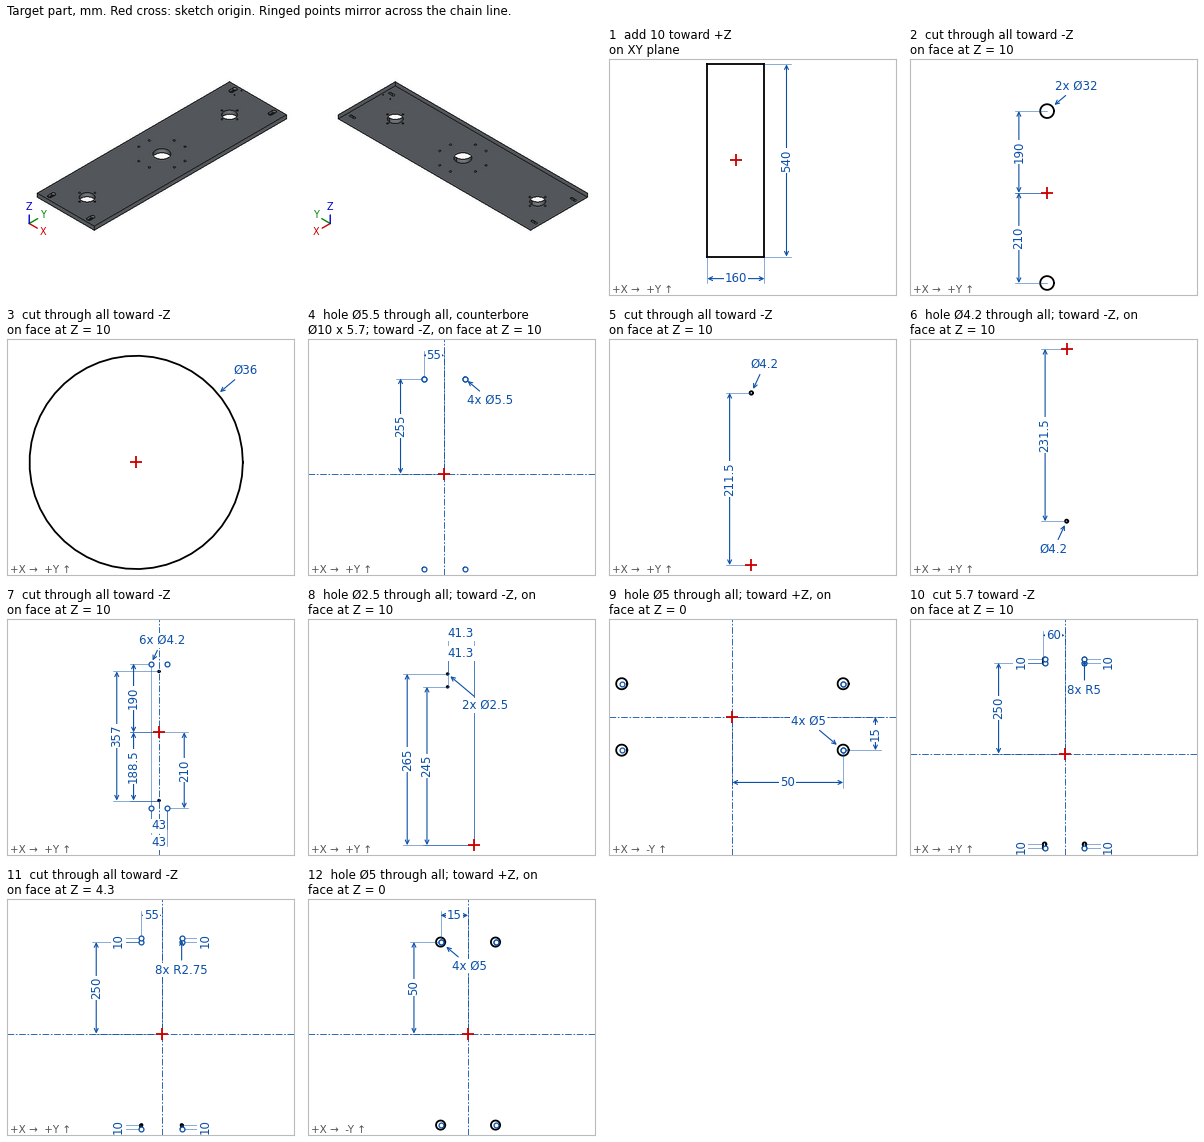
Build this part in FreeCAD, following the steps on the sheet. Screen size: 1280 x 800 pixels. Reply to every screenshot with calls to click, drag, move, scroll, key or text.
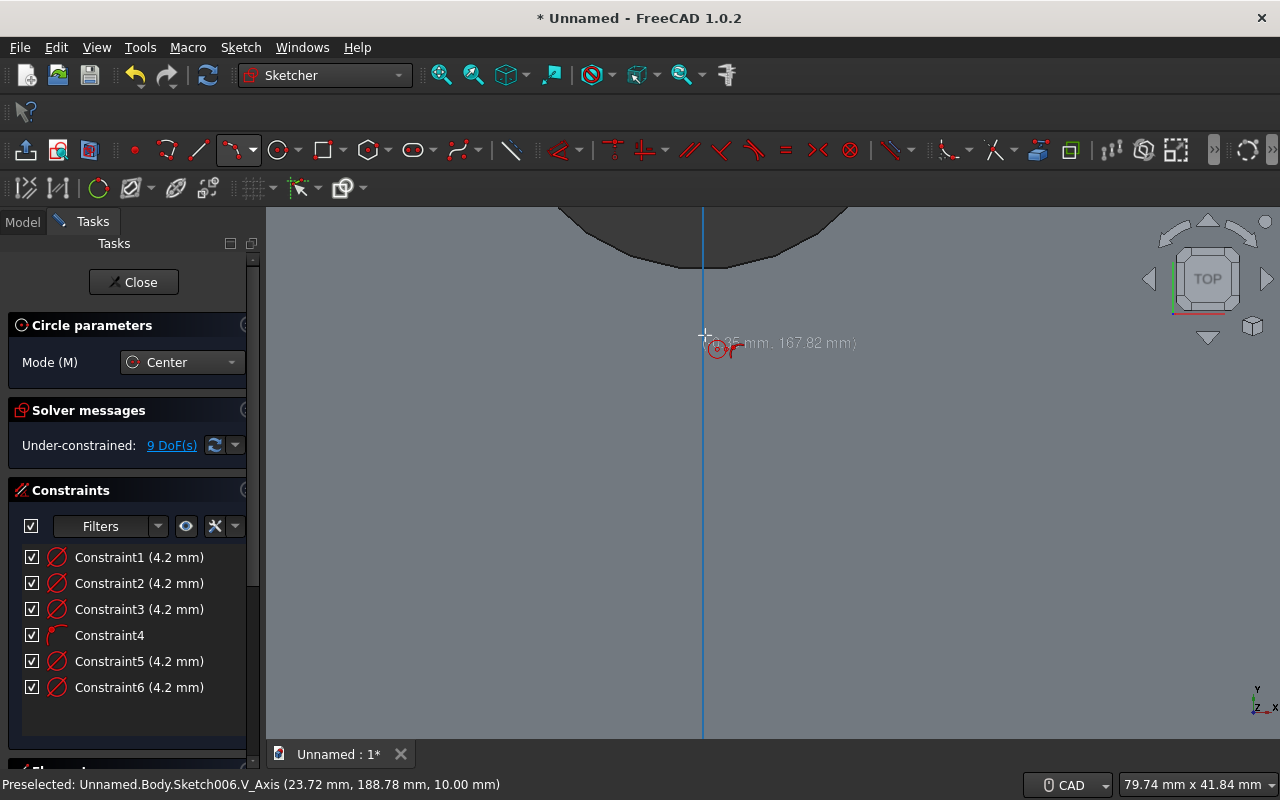
scroll(705, 335, down, 14)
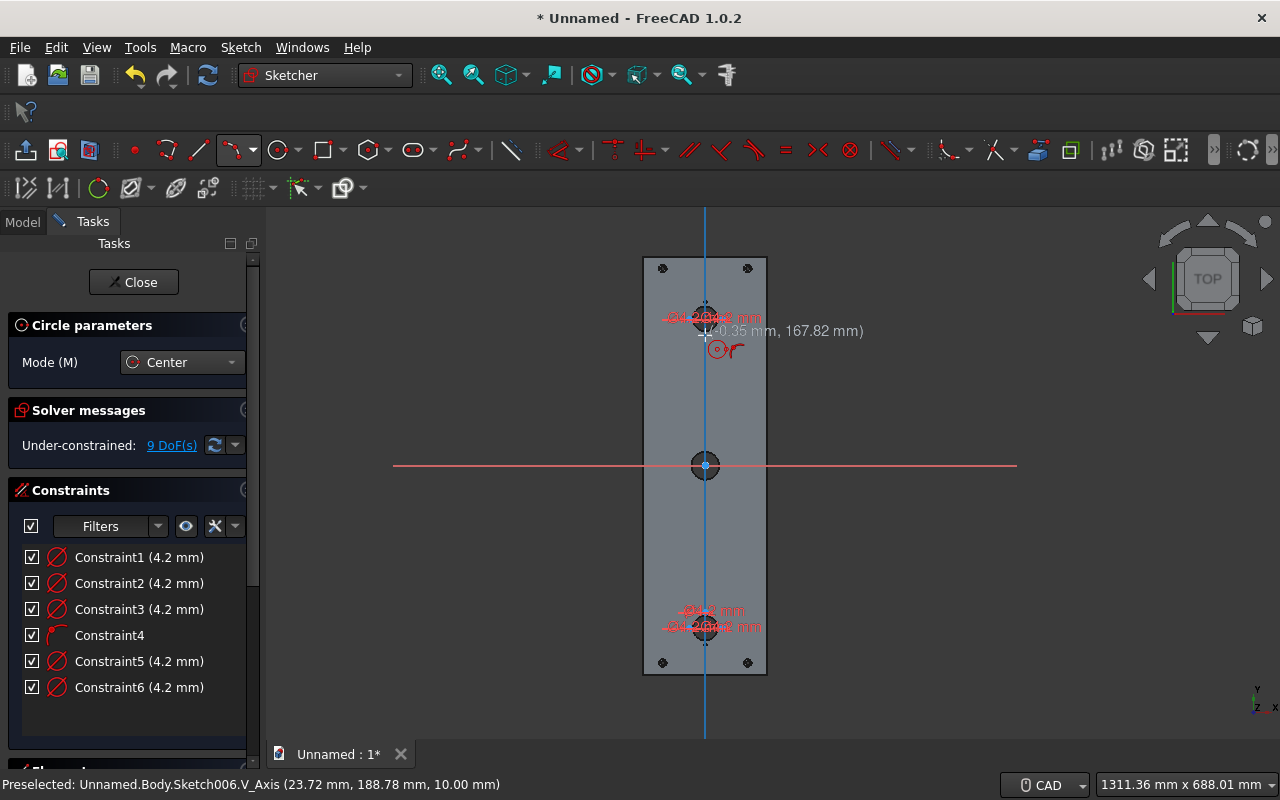
click(705, 335)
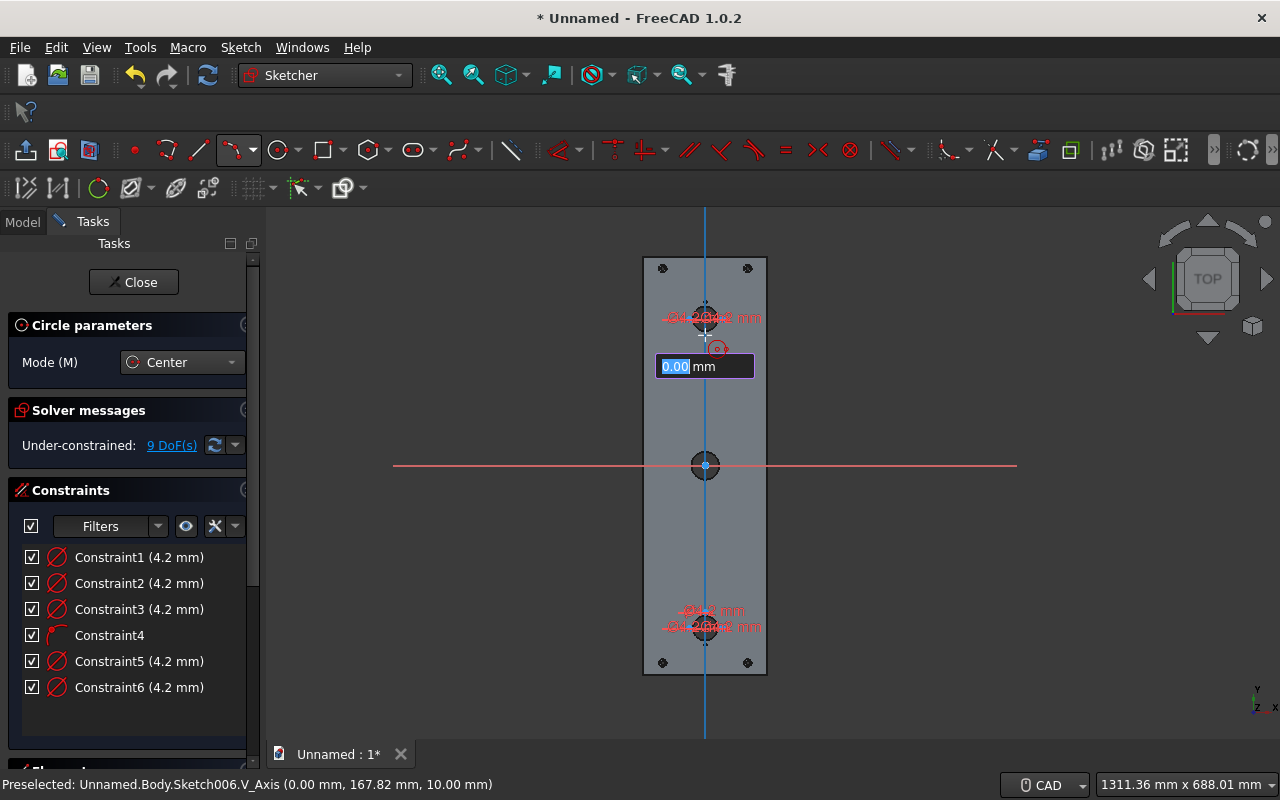
scroll(707, 335, up, 12)
move(700, 332)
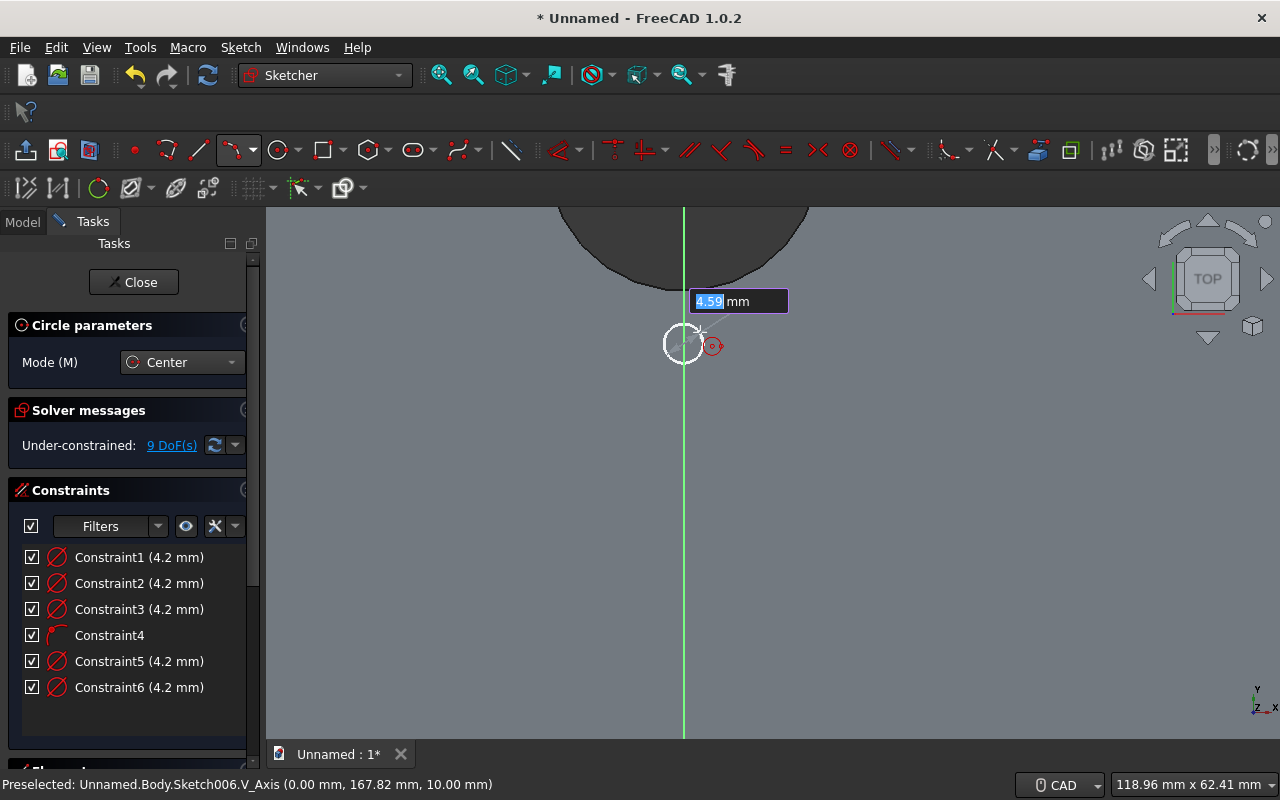
text(4.2)
key(Return)
key(Escape)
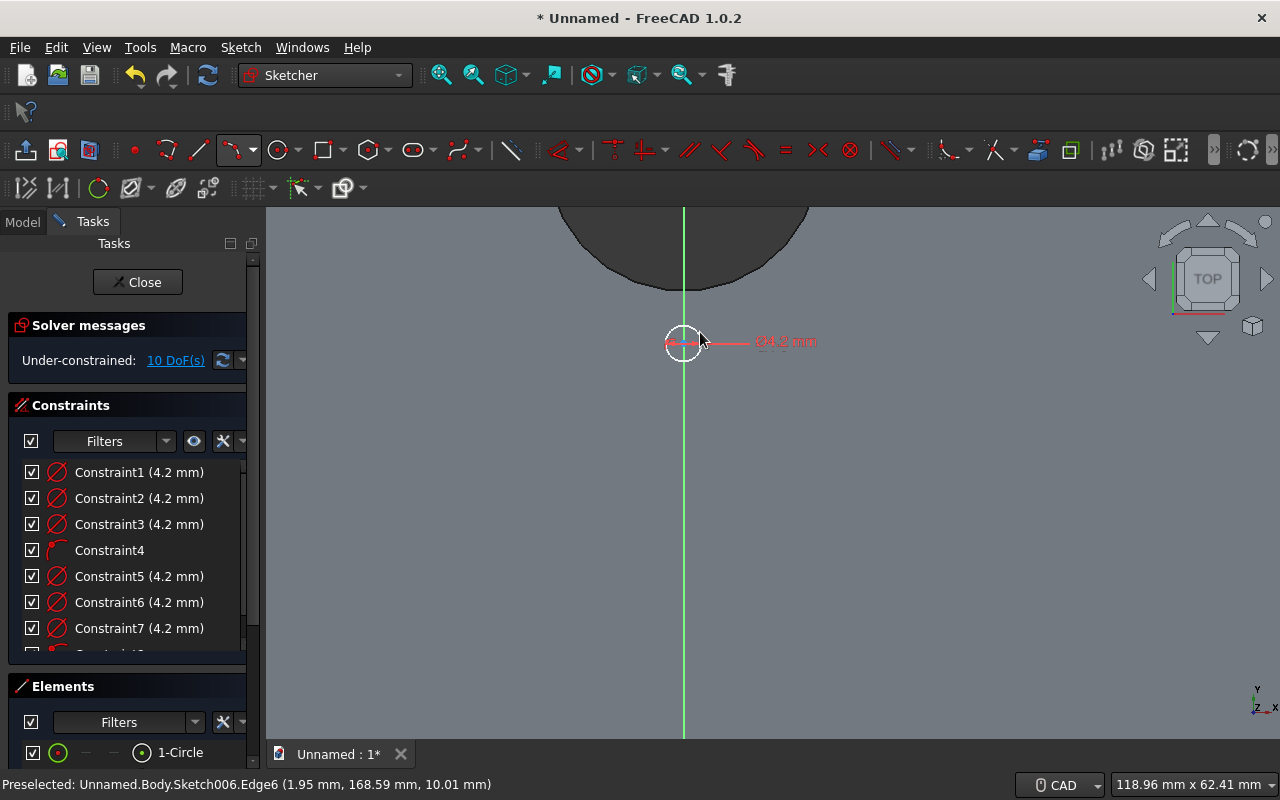
scroll(707, 335, down, 12)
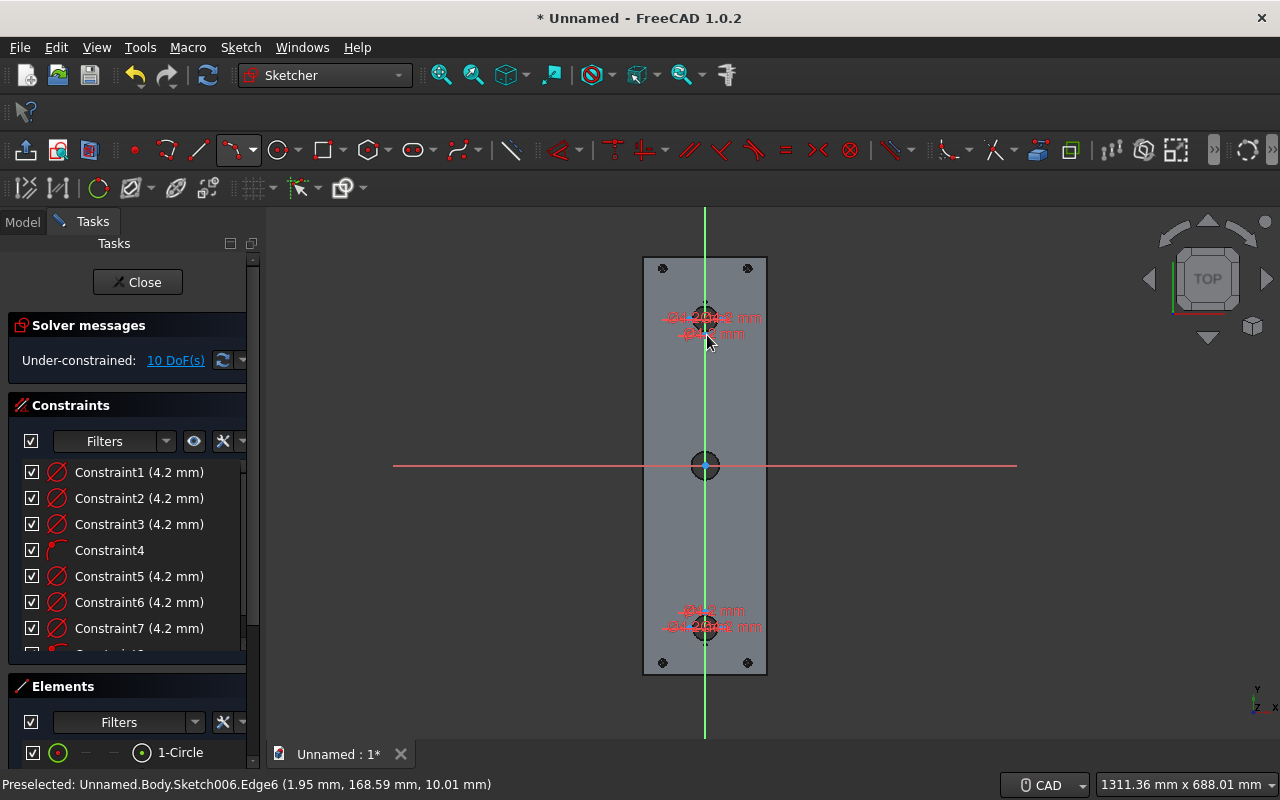
click(722, 629)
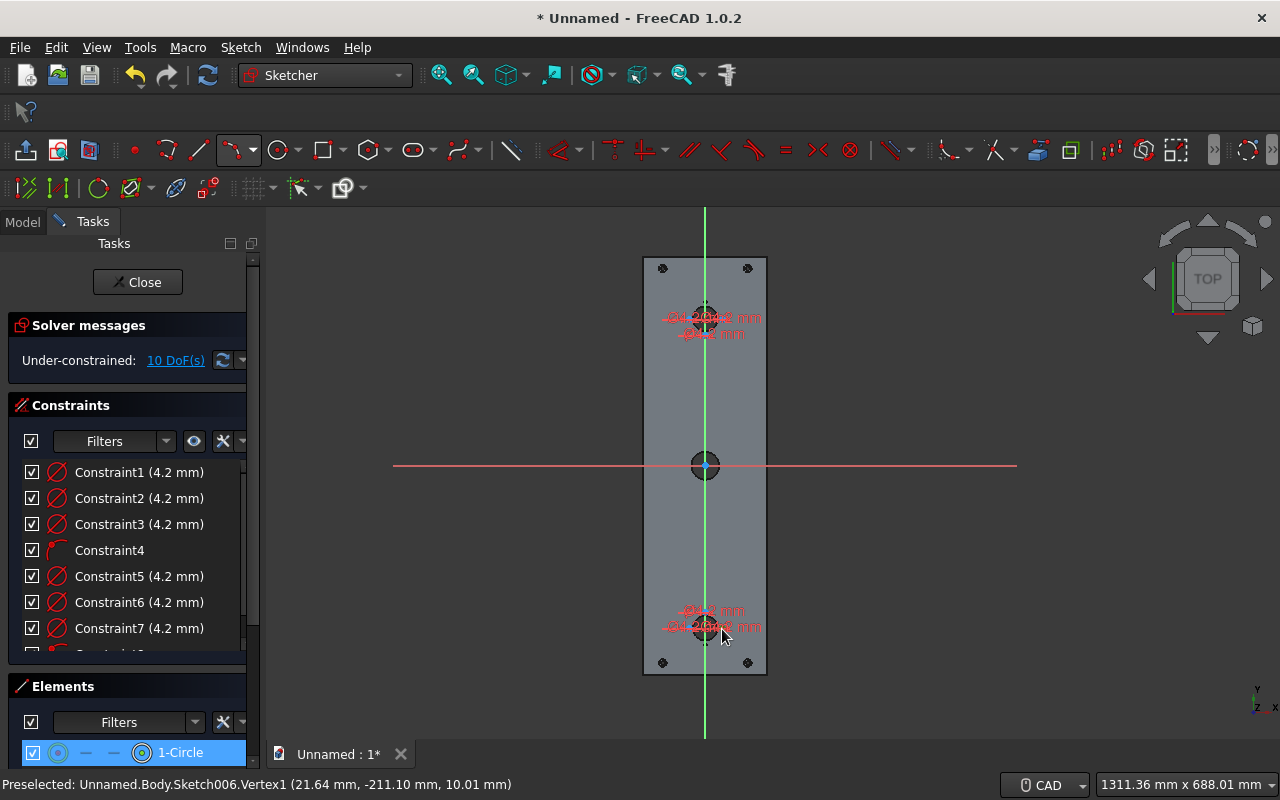
click(689, 629)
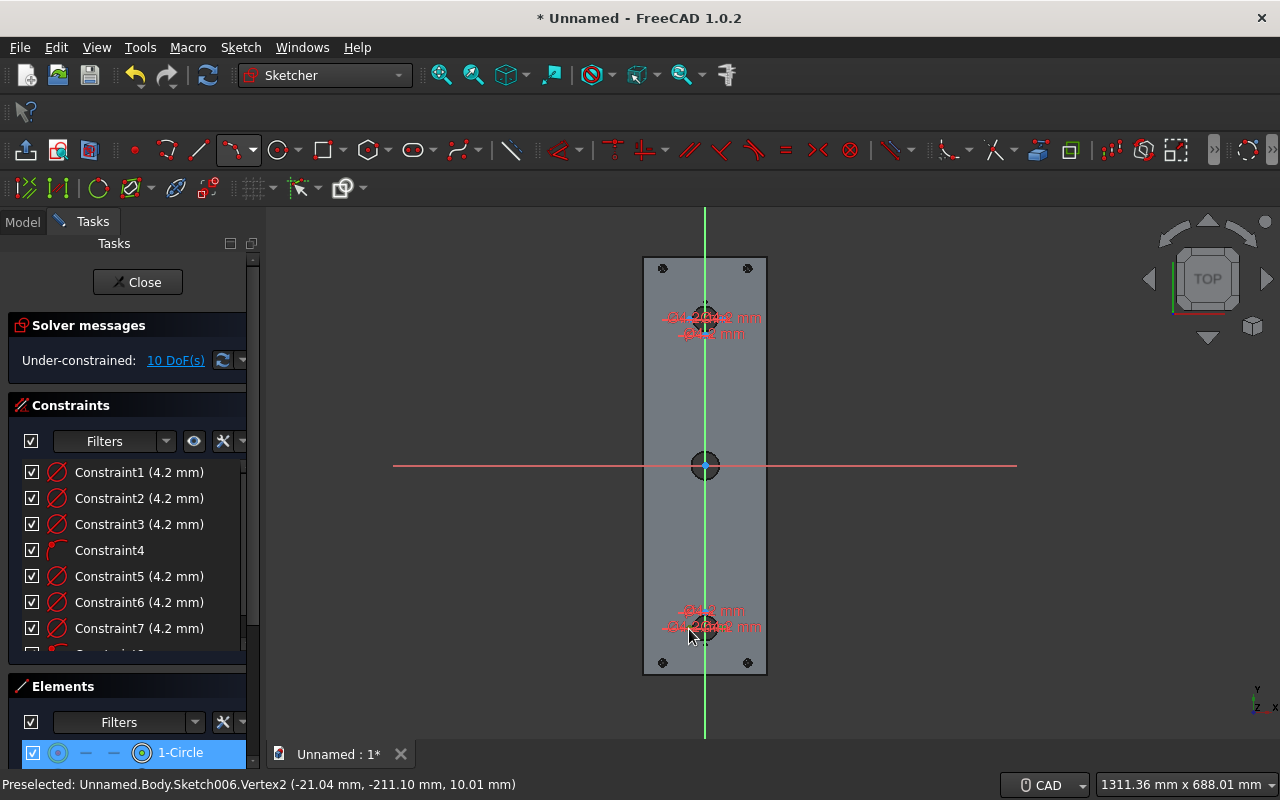
click(705, 677)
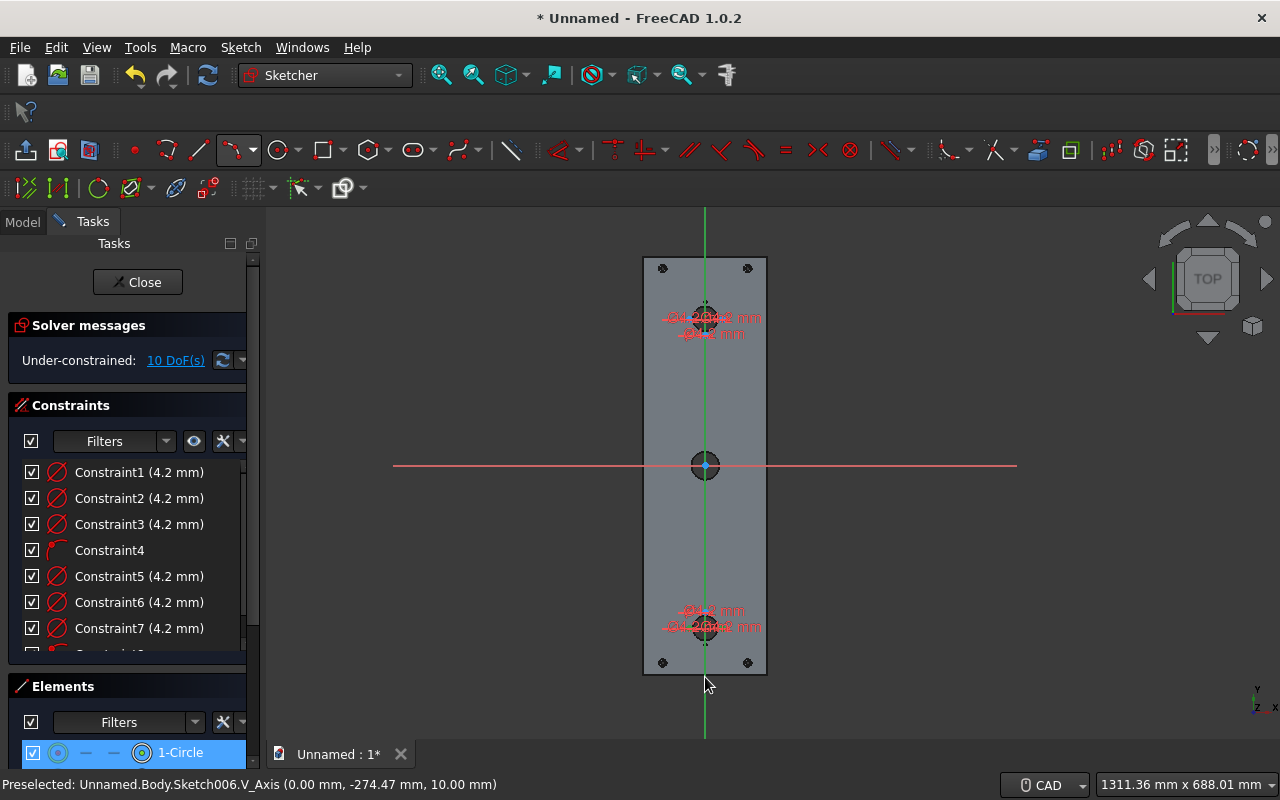
click(818, 150)